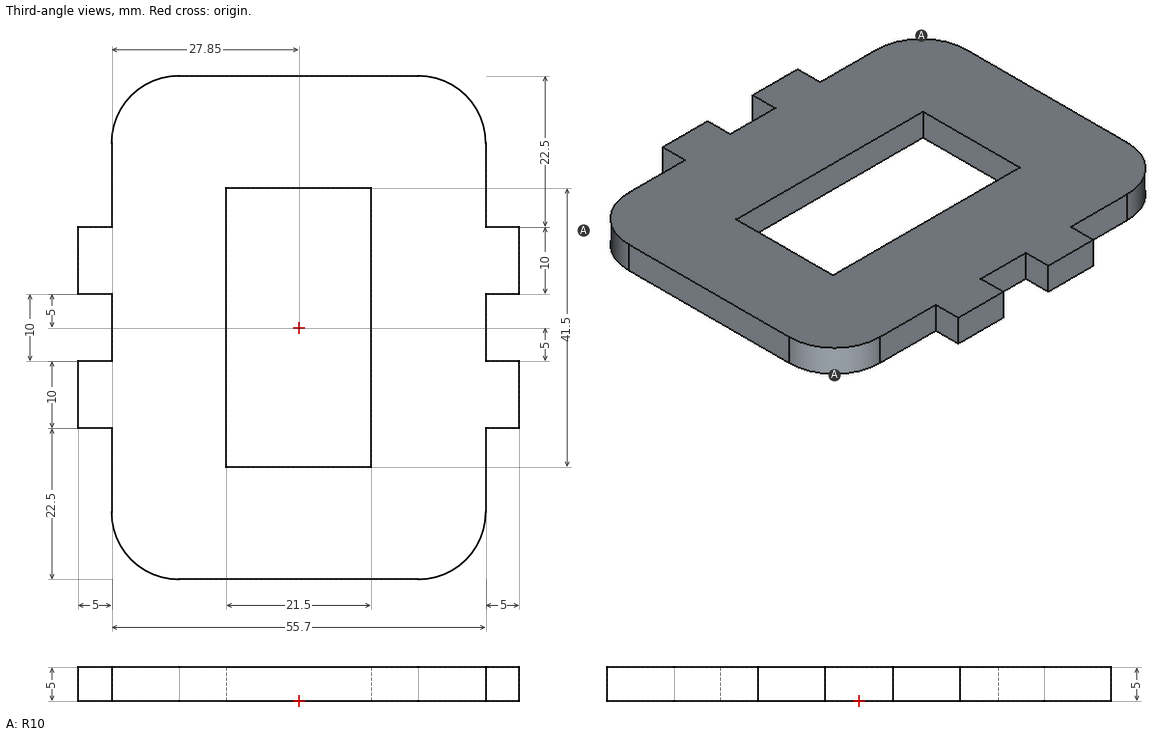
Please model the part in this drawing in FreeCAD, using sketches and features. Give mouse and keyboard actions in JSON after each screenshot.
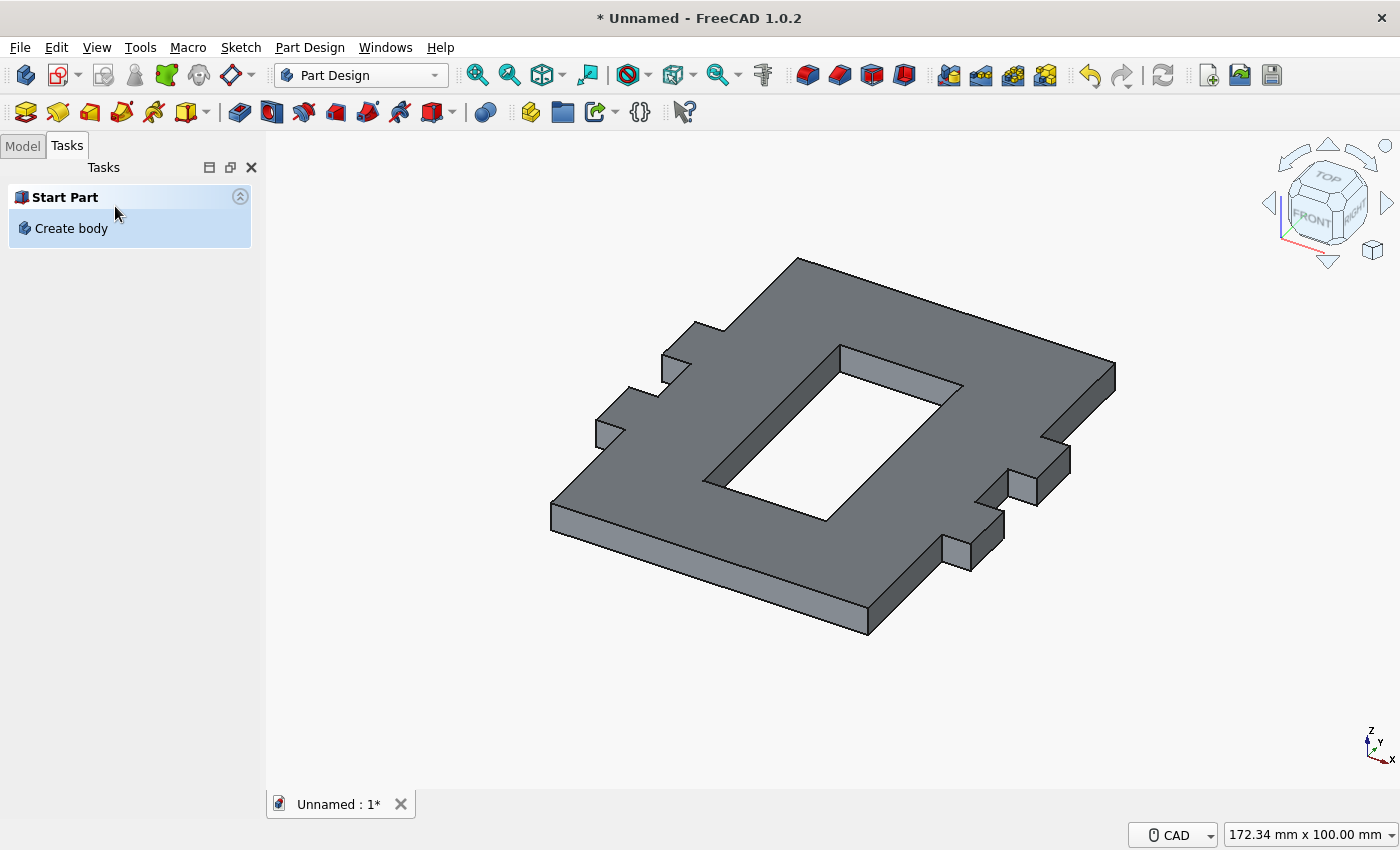
{"action": "left_click", "coordinate": [868, 621]}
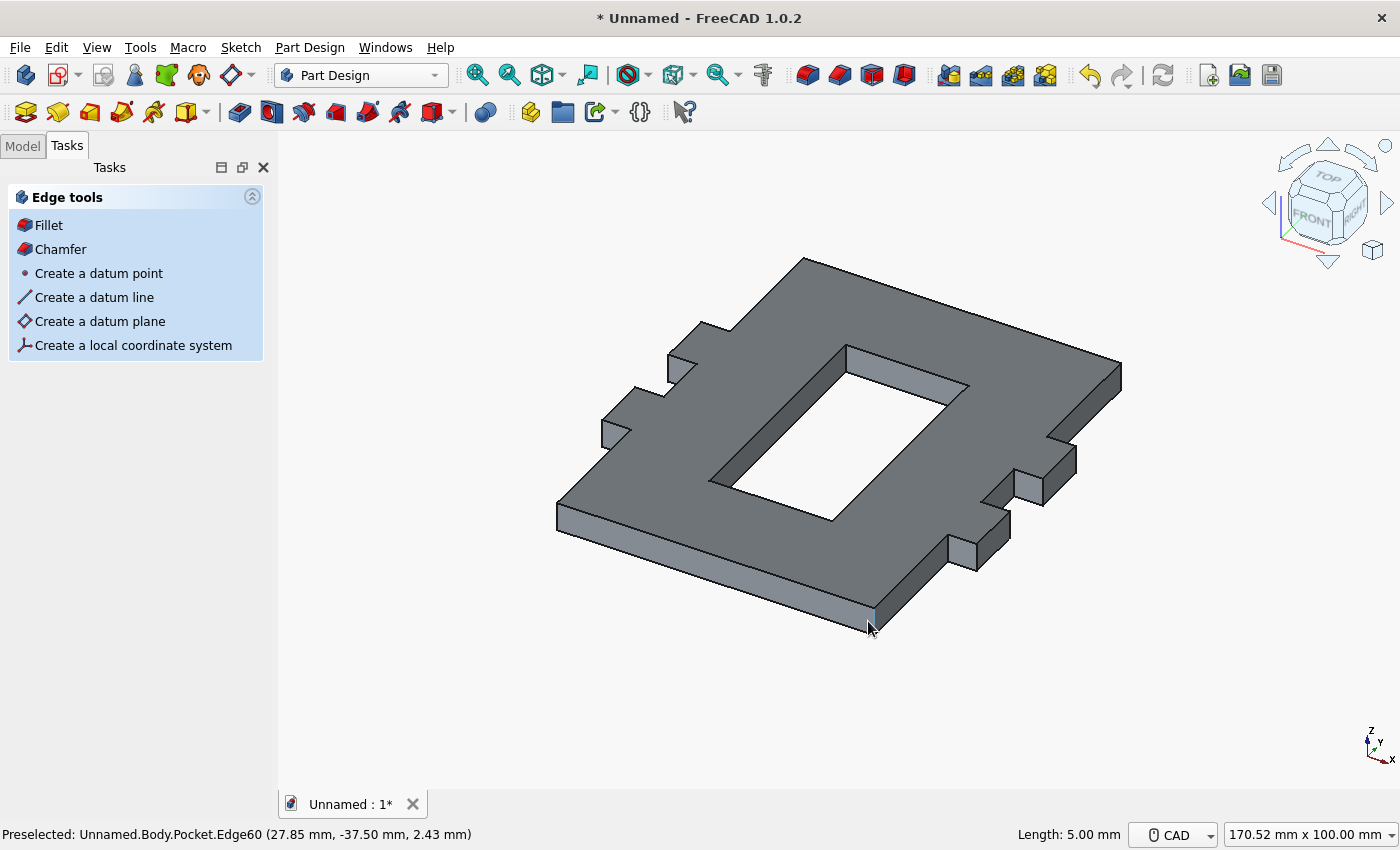
{"action": "key", "text": "0"}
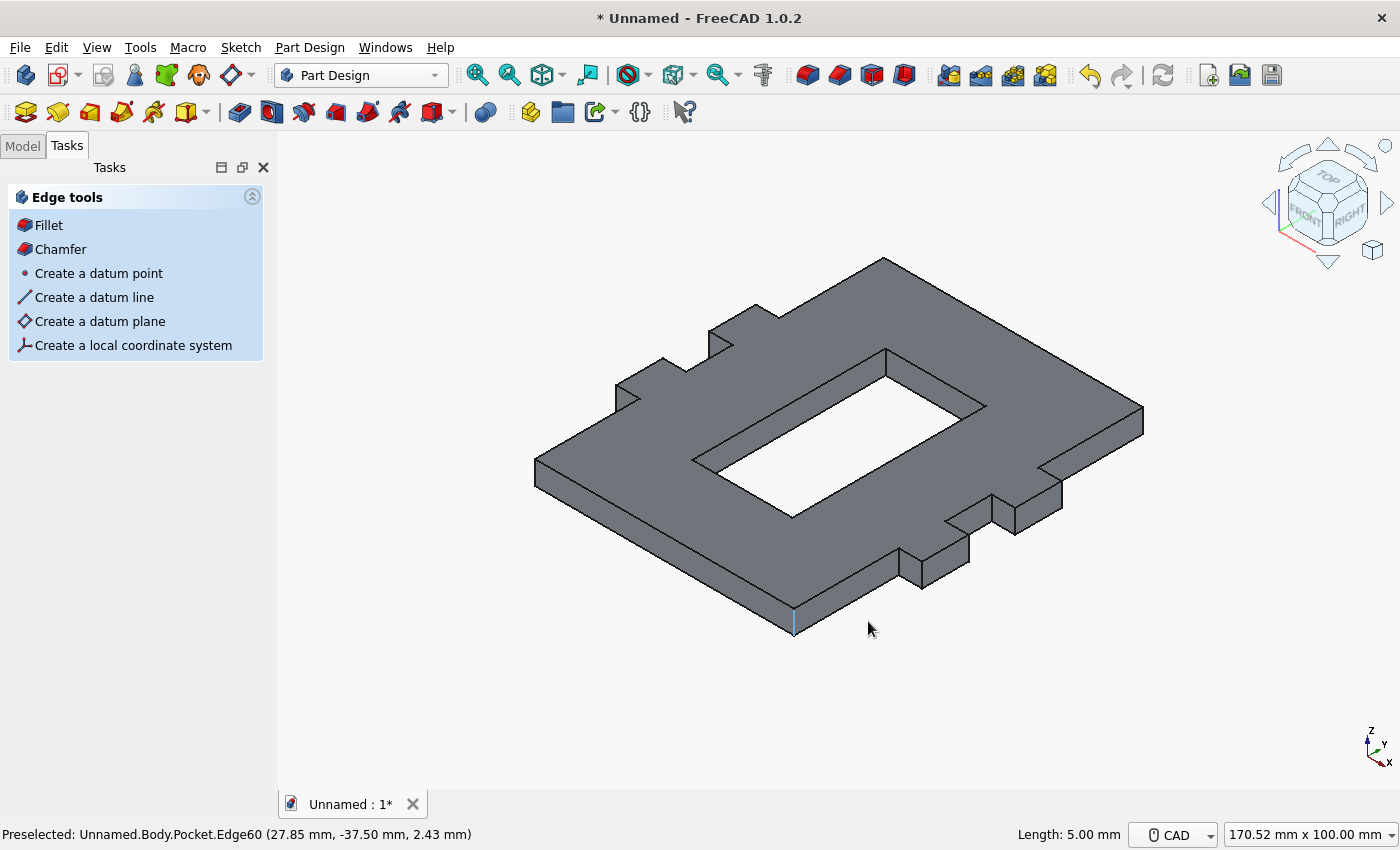
{"action": "key", "text": "2"}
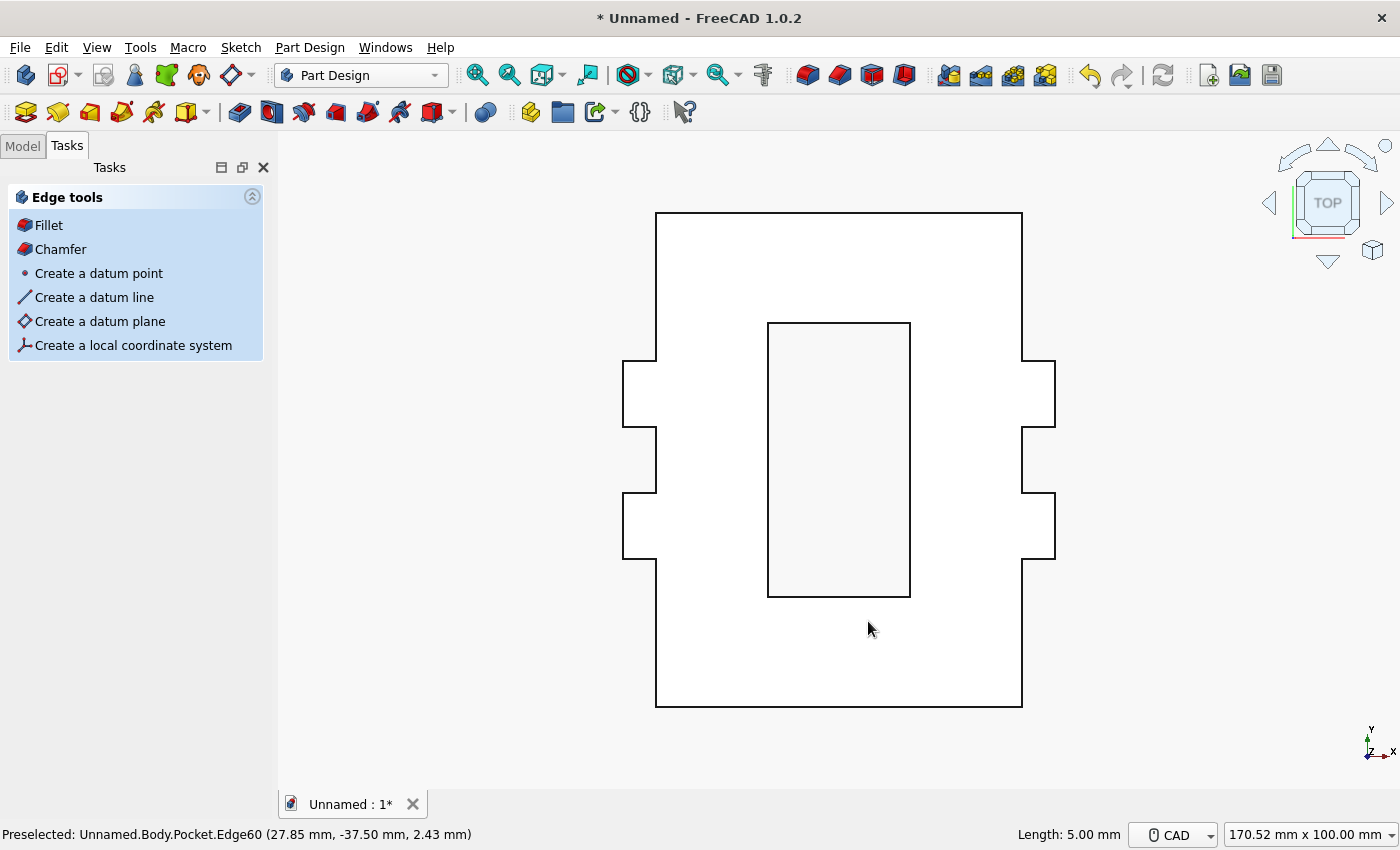
{"action": "key", "text": "1"}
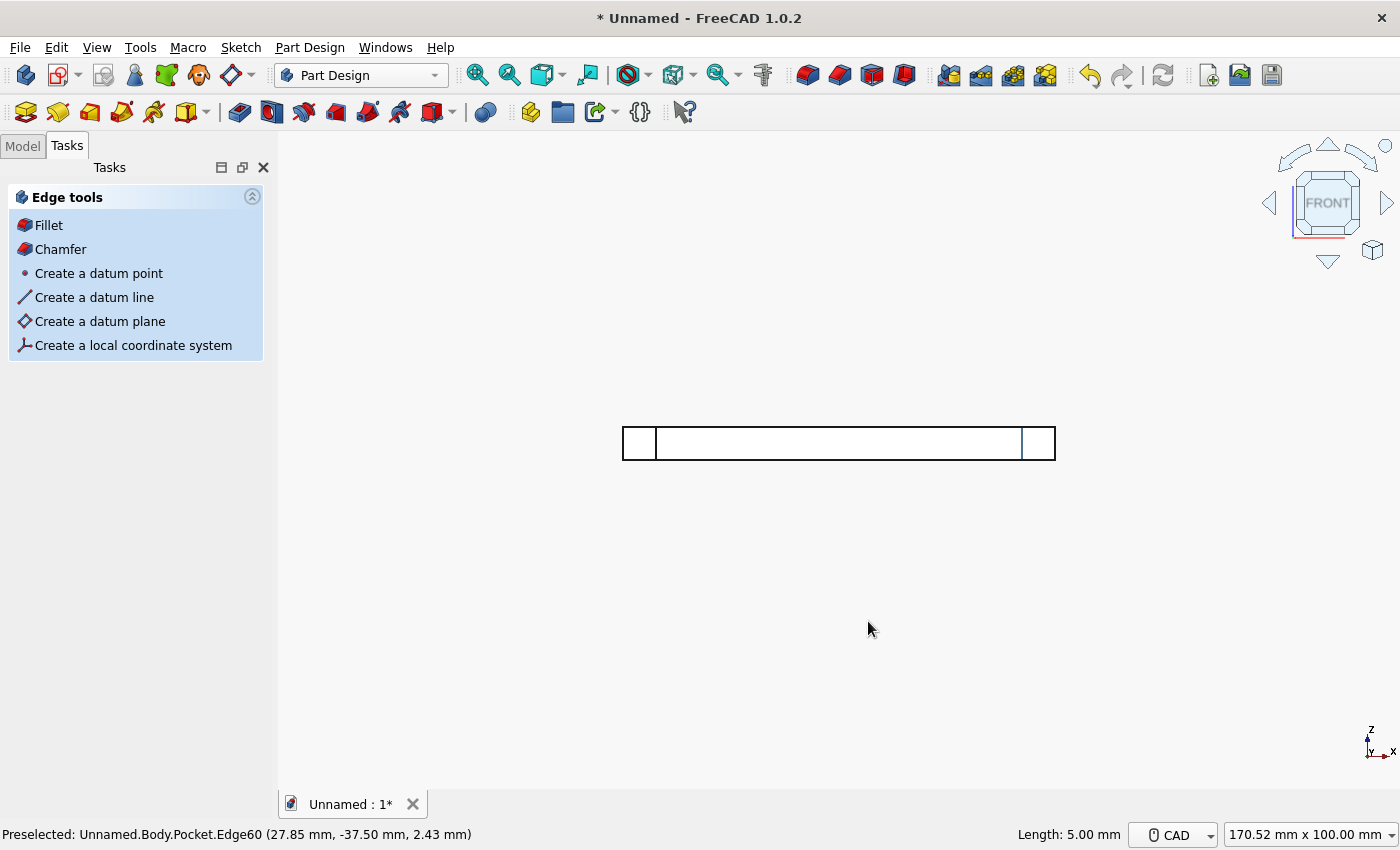
{"action": "left_click", "coordinate": [478, 76]}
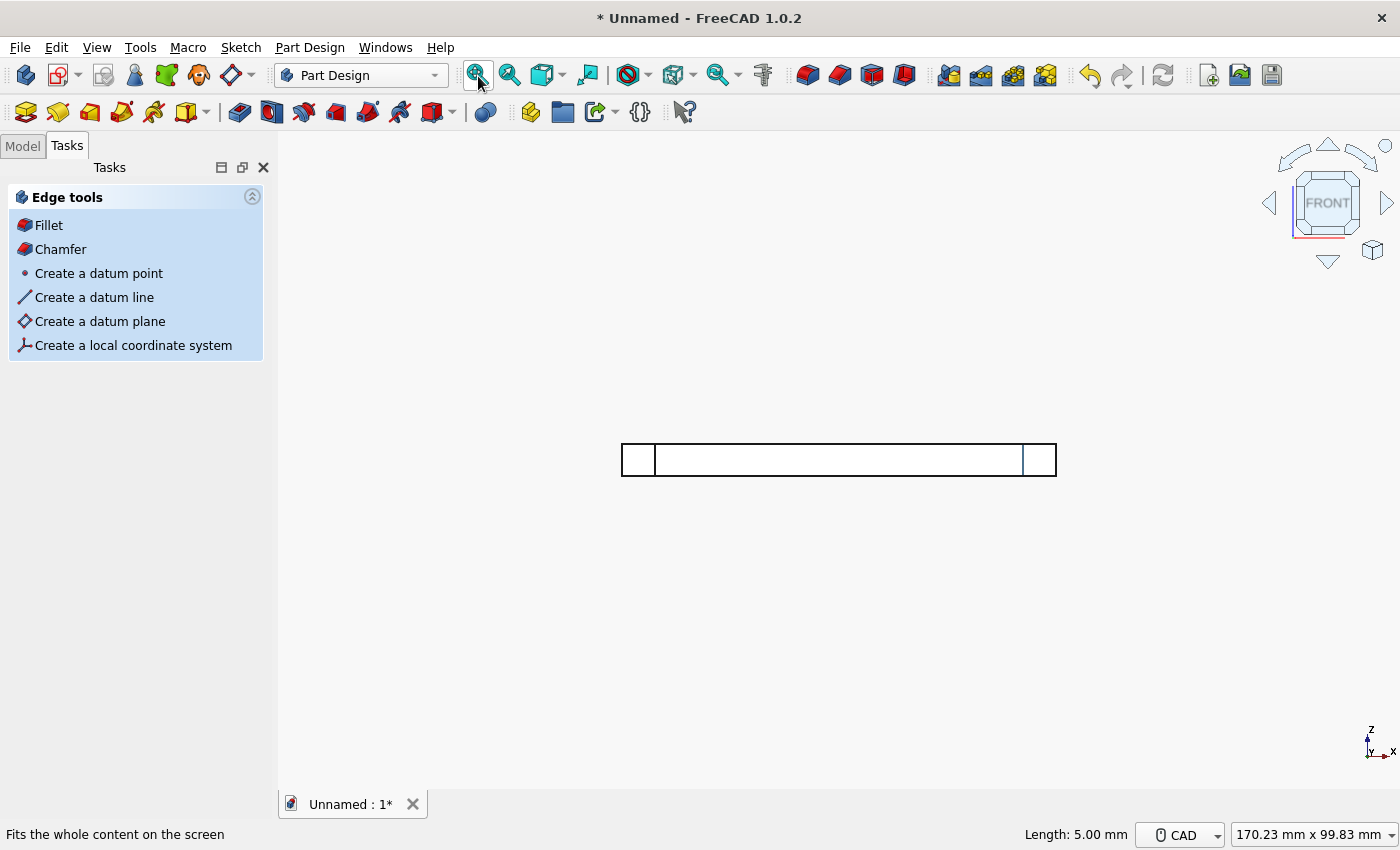
{"action": "left_click", "coordinate": [655, 459], "text": "ctrl"}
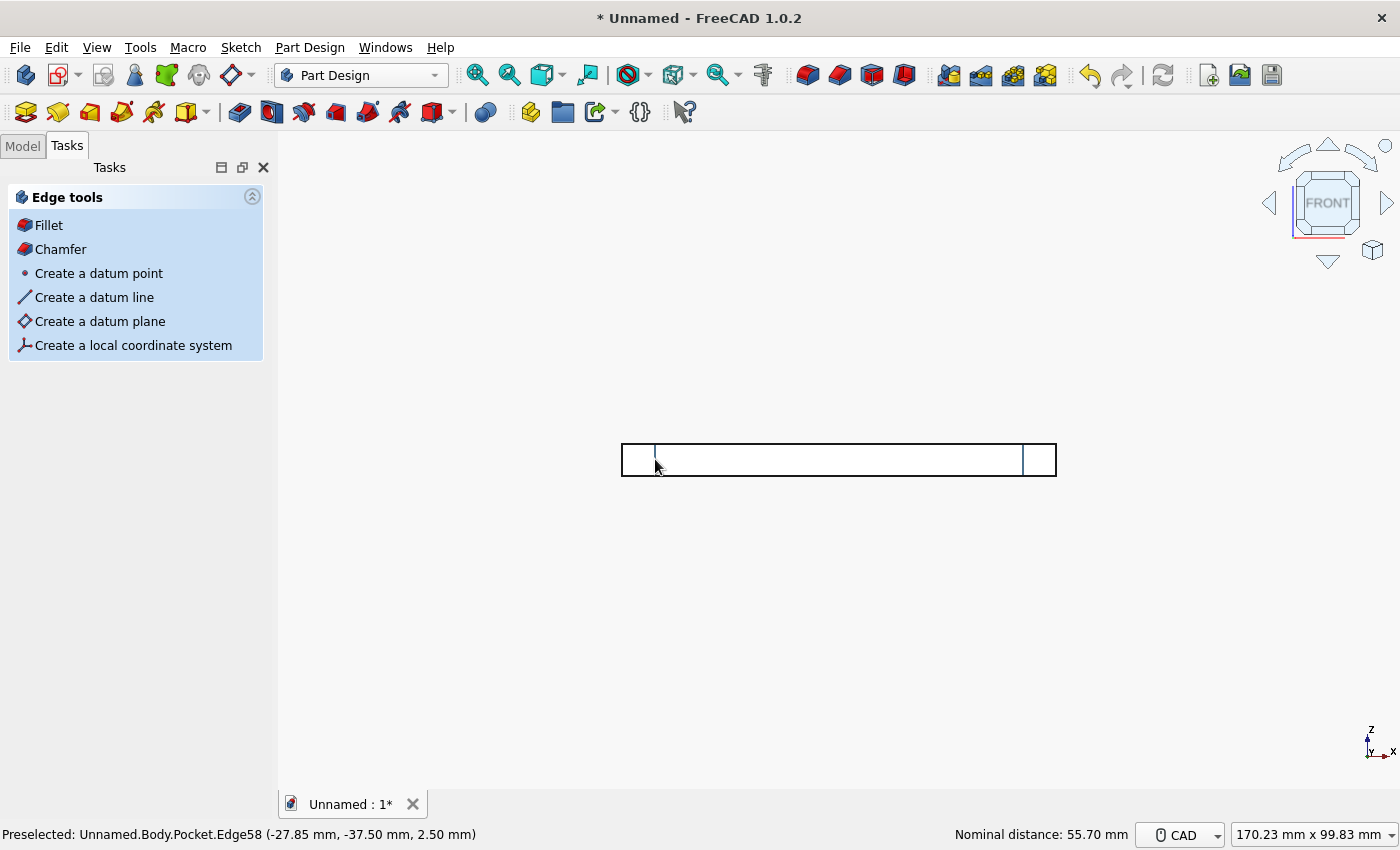
{"action": "key", "text": "3"}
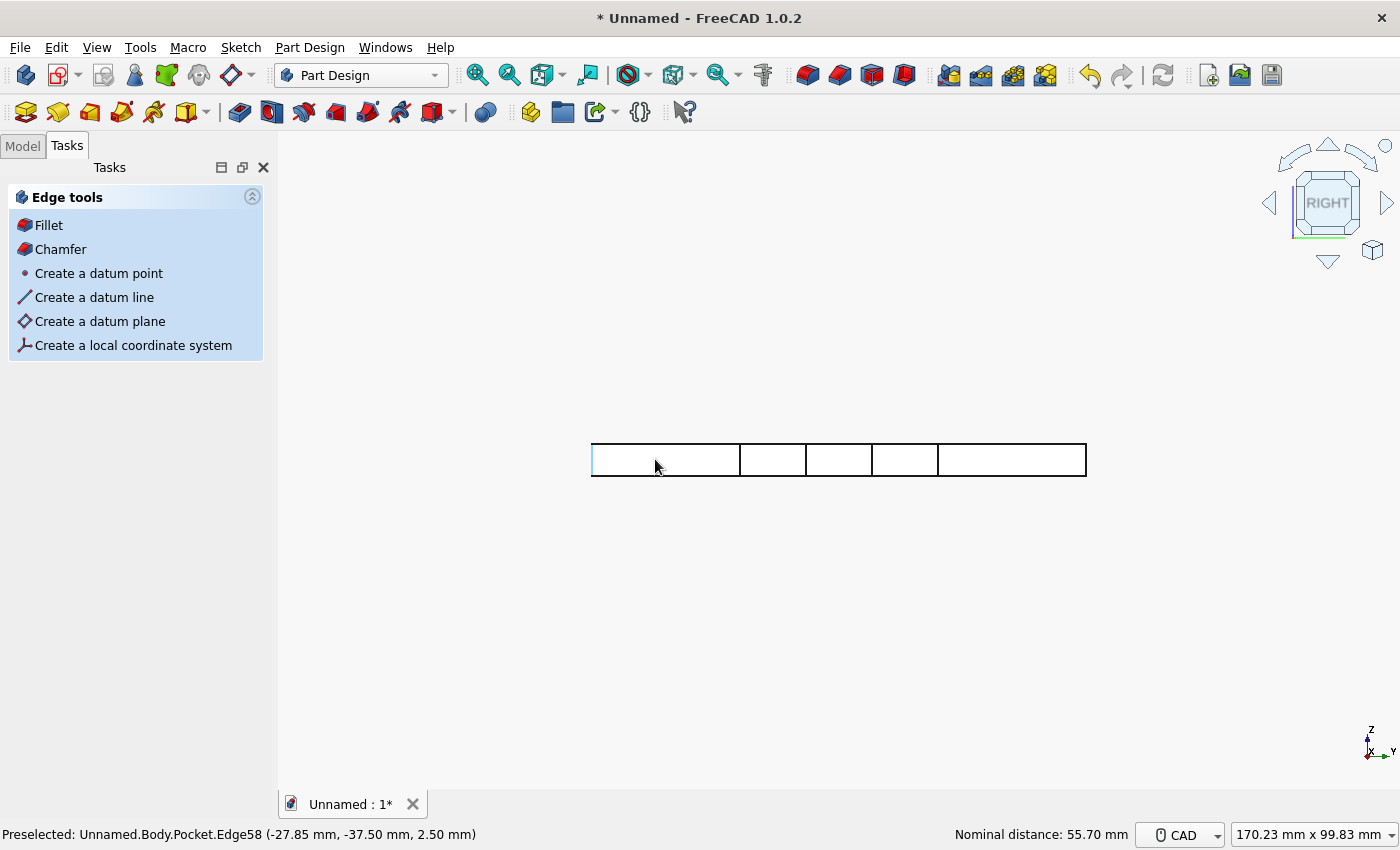
{"action": "left_click", "coordinate": [478, 76]}